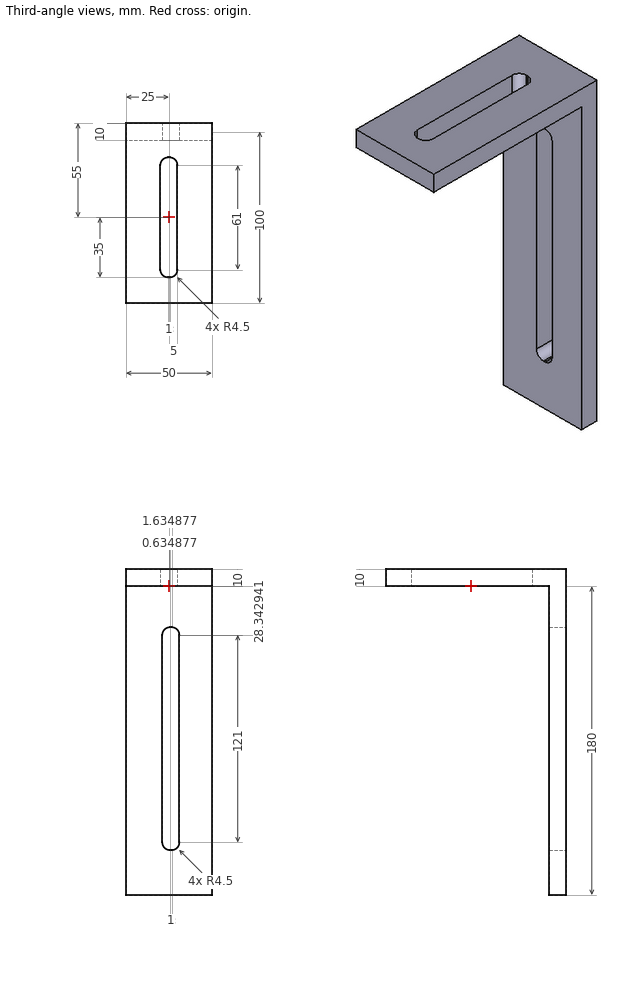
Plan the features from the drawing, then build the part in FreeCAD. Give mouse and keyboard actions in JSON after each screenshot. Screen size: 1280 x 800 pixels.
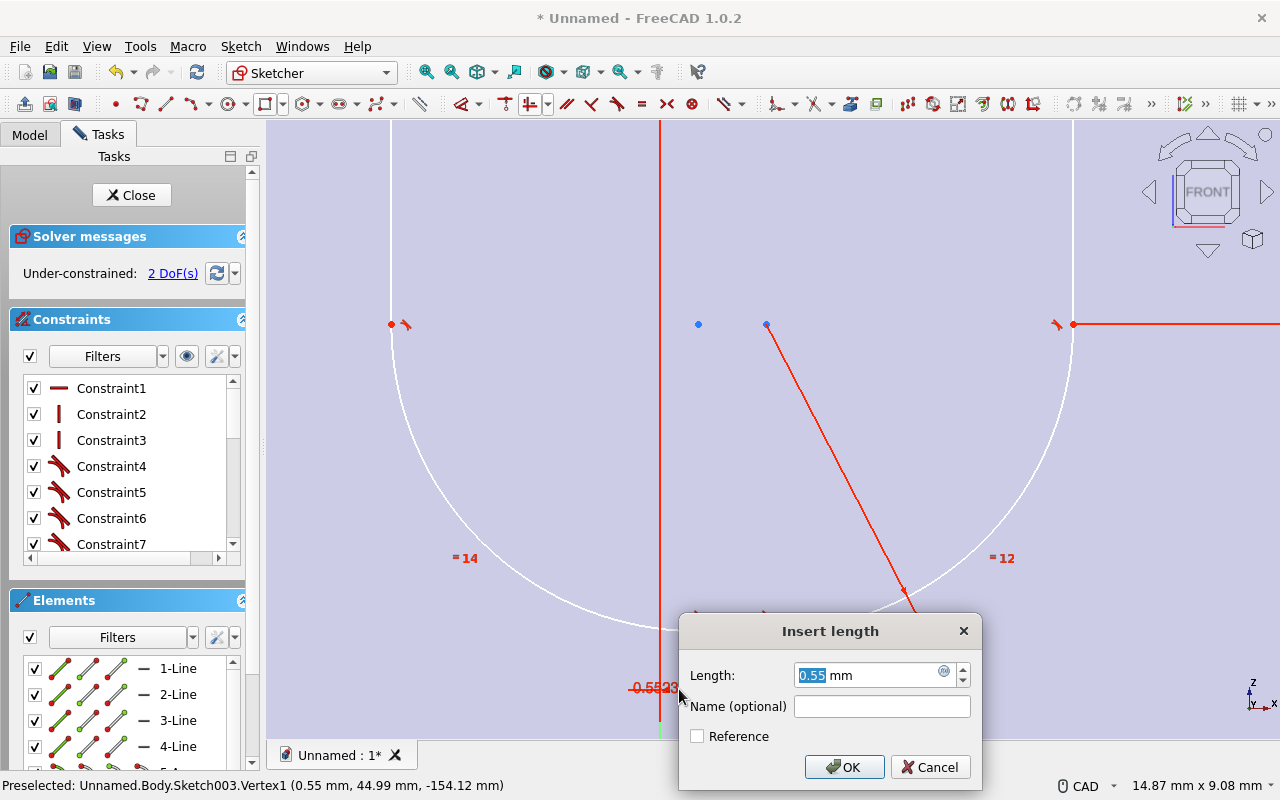
{"action": "type", "text": "0.634877"}
{"action": "key", "text": "Return"}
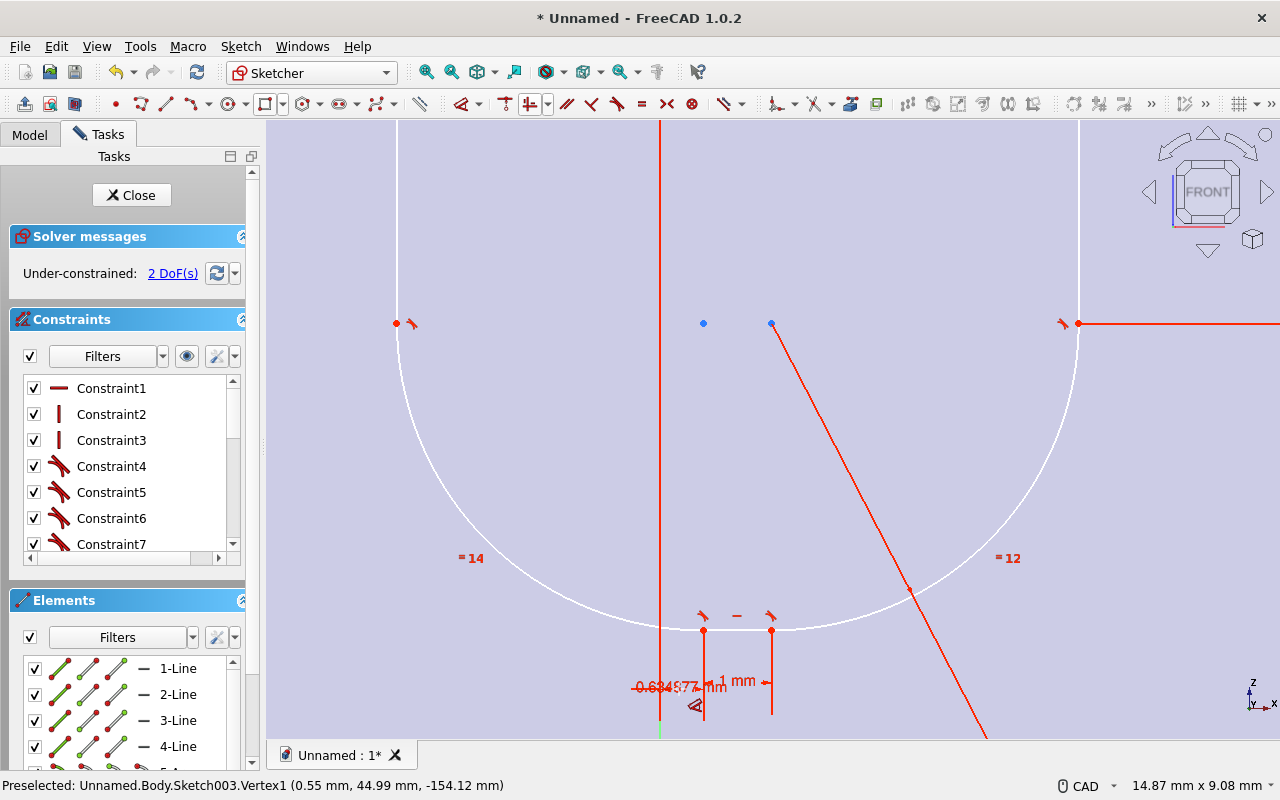
{"action": "scroll", "coordinate": [703, 645], "scroll_direction": "down", "scroll_amount": 16}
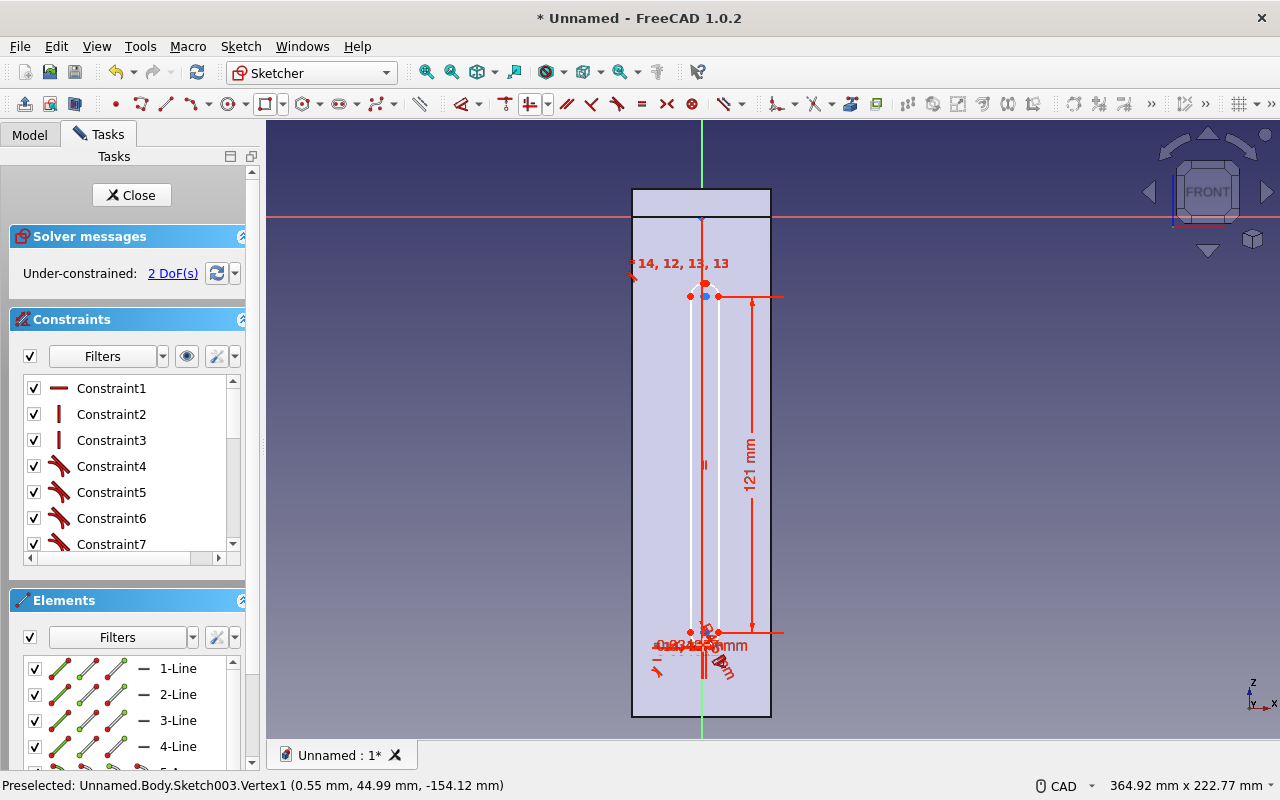
{"action": "scroll", "coordinate": [706, 284], "scroll_direction": "up", "scroll_amount": 11}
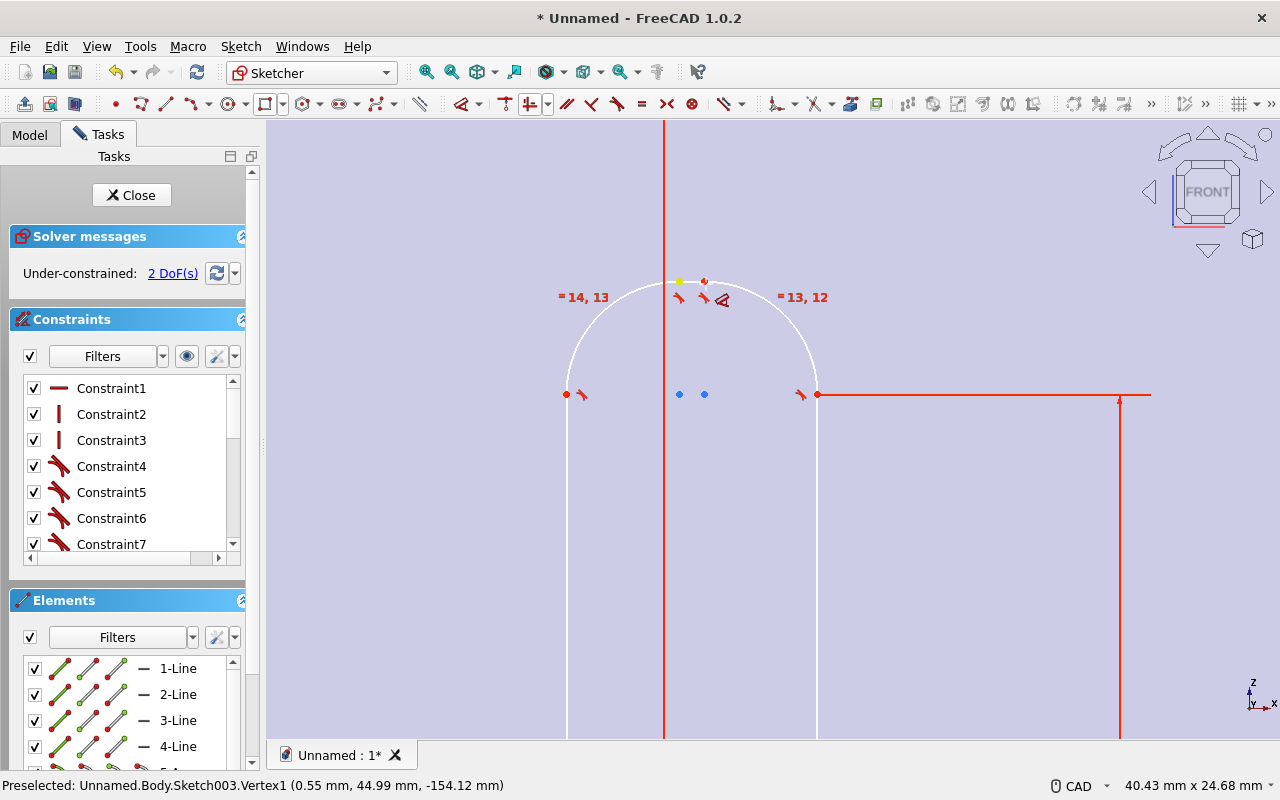
{"action": "left_click", "coordinate": [705, 282]}
{"action": "left_click", "coordinate": [684, 316]}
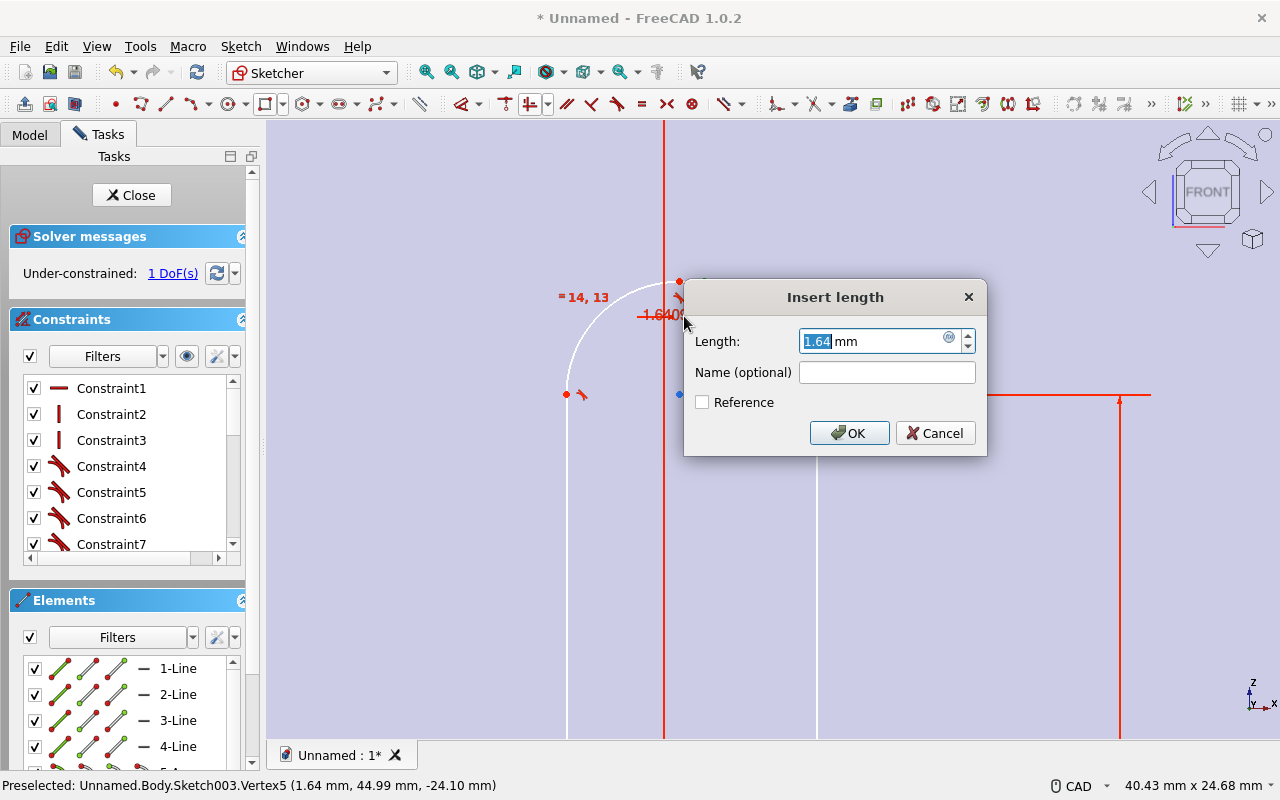
{"action": "type", "text": "1.634877"}
{"action": "key", "text": "Return"}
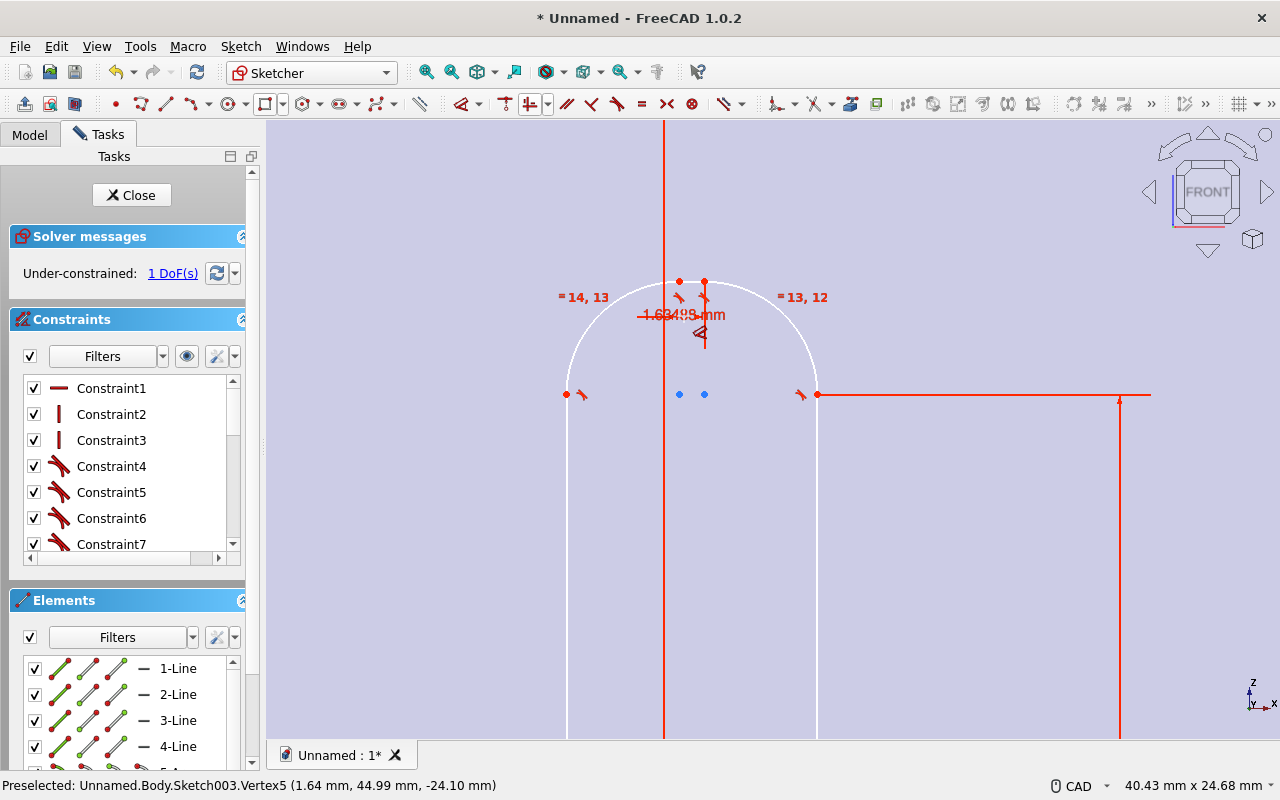
{"action": "scroll", "coordinate": [706, 283], "scroll_direction": "down", "scroll_amount": 11}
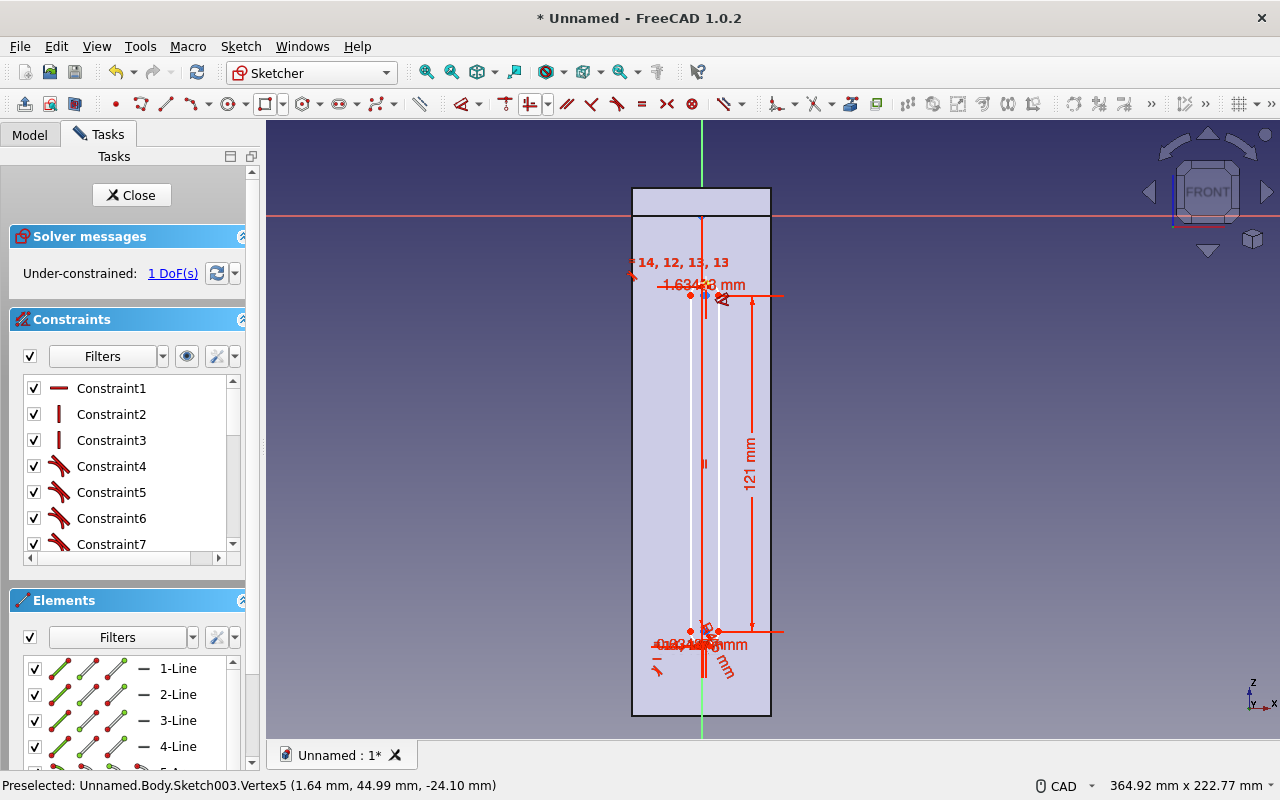
{"action": "left_click", "coordinate": [719, 296]}
{"action": "left_click", "coordinate": [753, 256]}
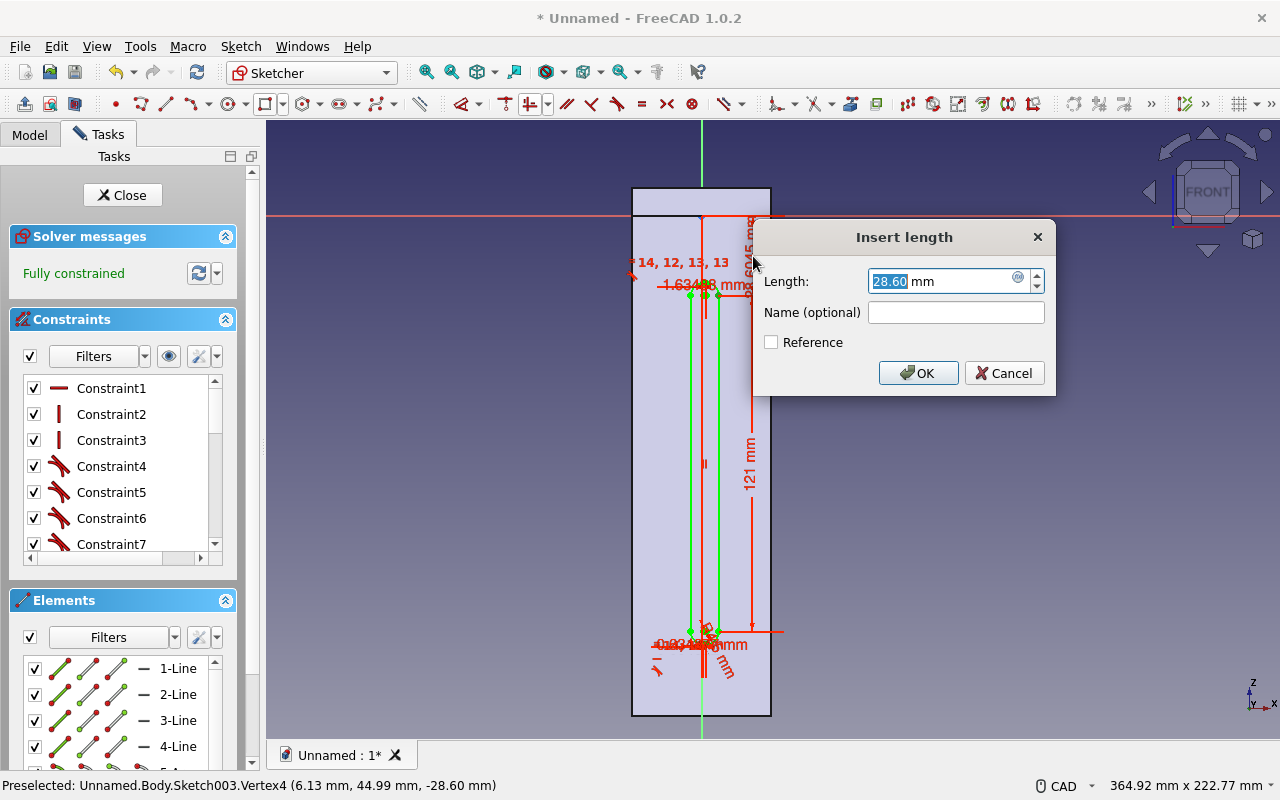
{"action": "type", "text": "28.342941"}
{"action": "key", "text": "Return"}
{"action": "key", "text": "Escape"}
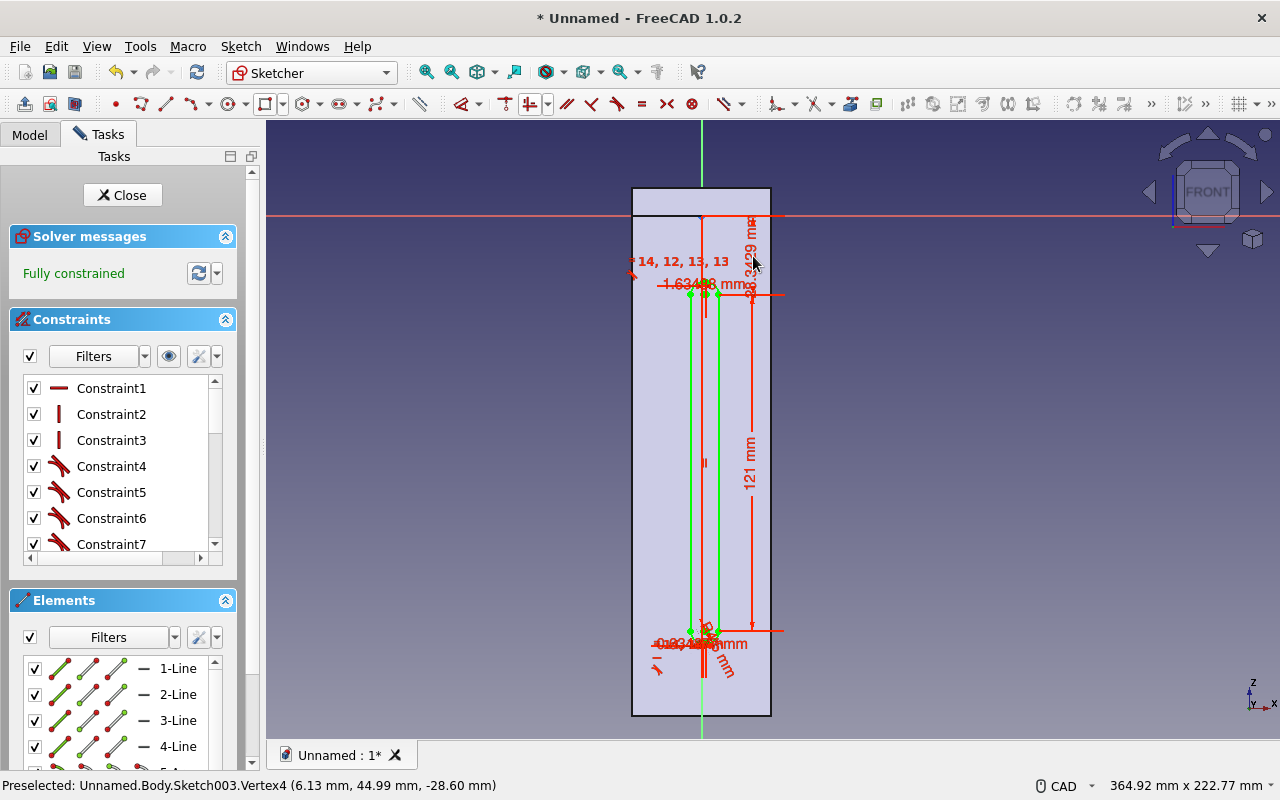
{"action": "left_click", "coordinate": [123, 195]}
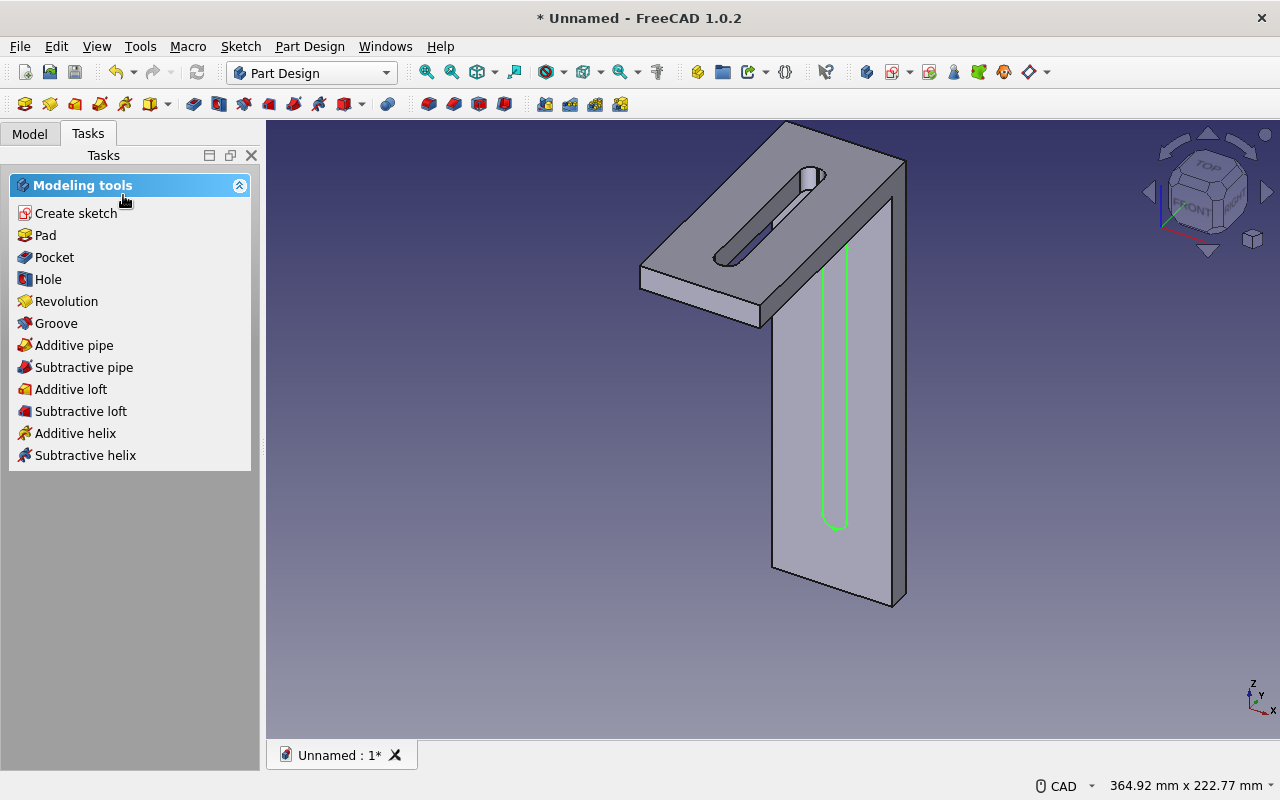
{"action": "left_click", "coordinate": [194, 104]}